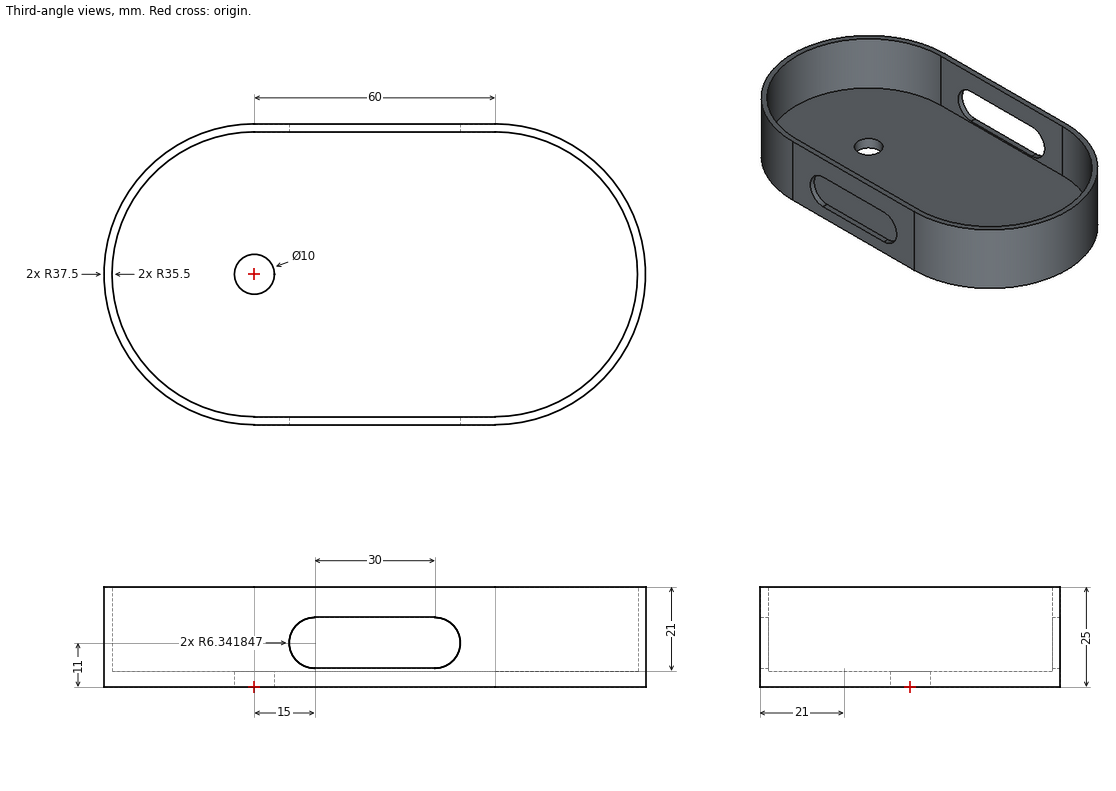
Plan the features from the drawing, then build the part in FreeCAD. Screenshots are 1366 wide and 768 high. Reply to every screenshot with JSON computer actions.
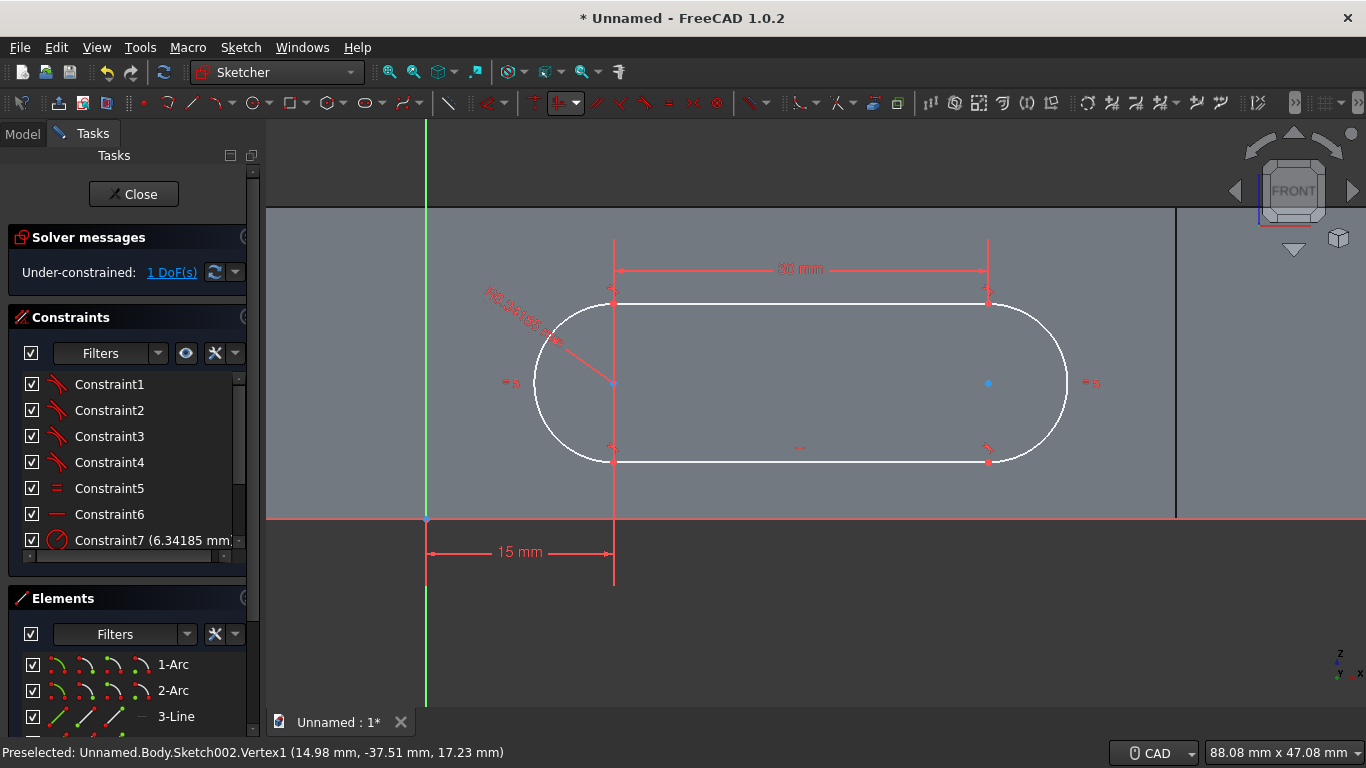
{"action": "left_click", "coordinate": [614, 383]}
{"action": "left_click", "coordinate": [392, 451]}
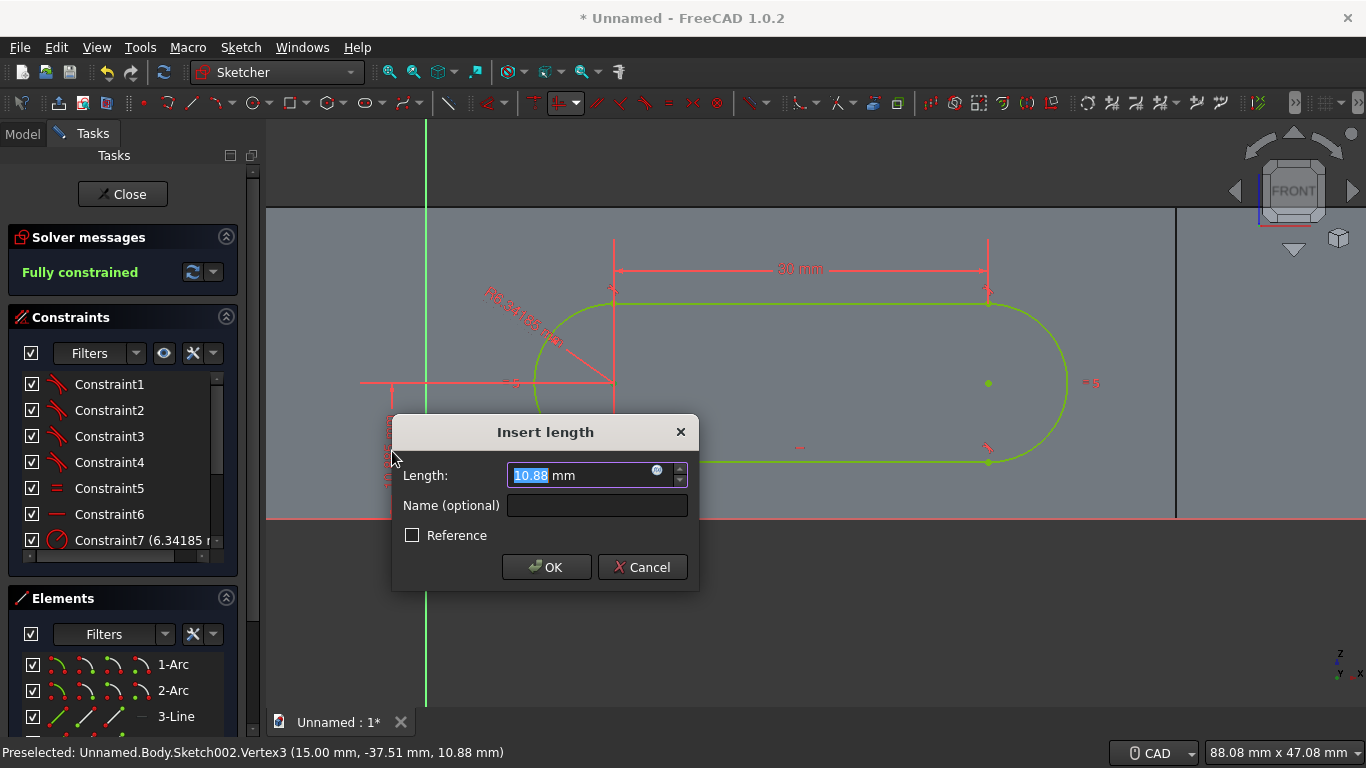
{"action": "type", "text": "11"}
{"action": "key", "text": "Return"}
{"action": "key", "text": "Escape"}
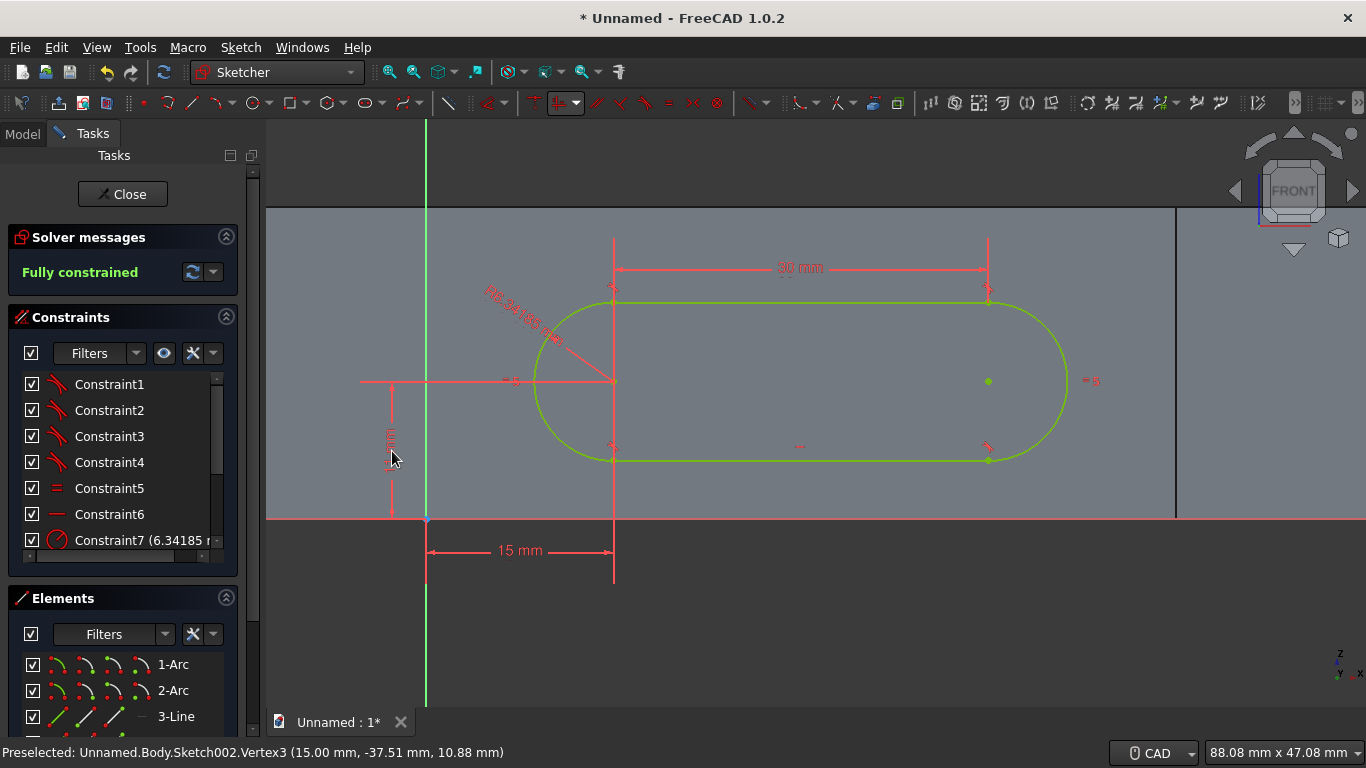
{"action": "left_click", "coordinate": [123, 194]}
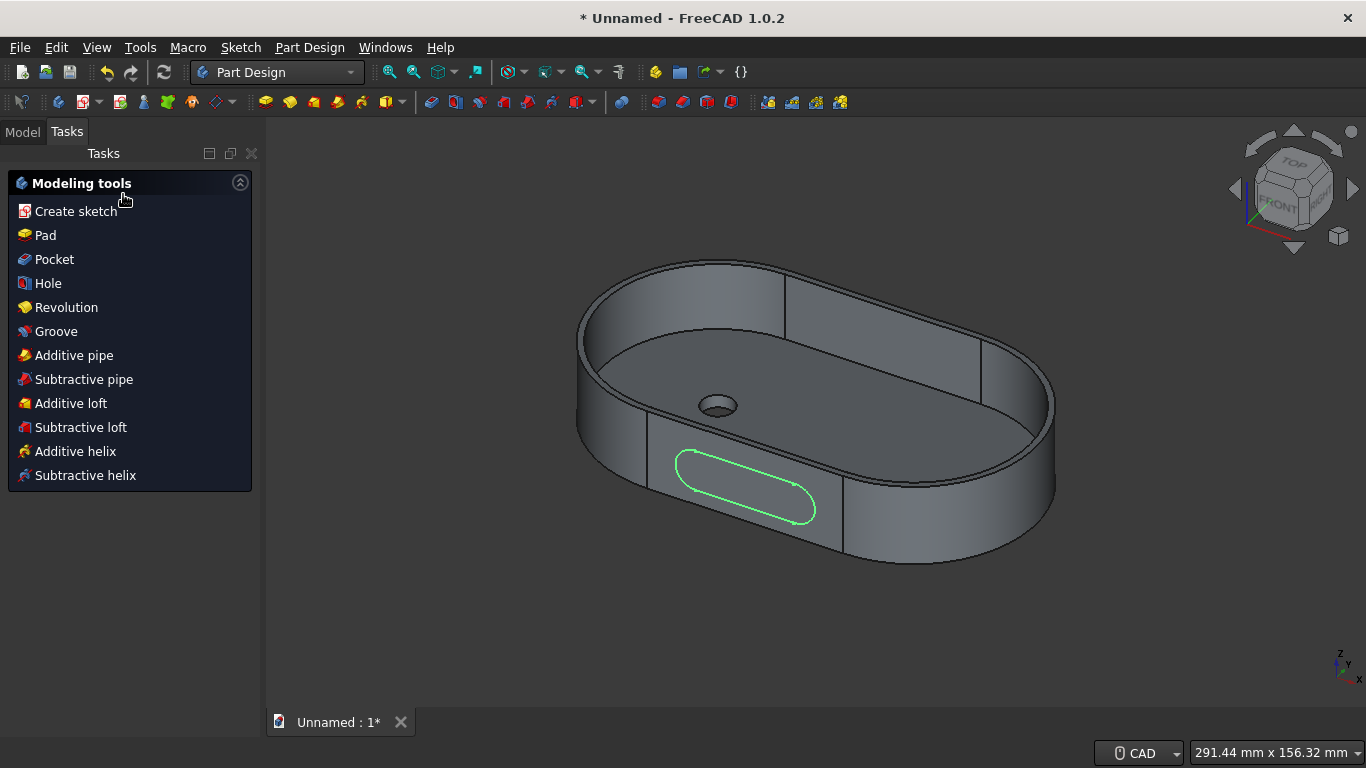
{"action": "left_click", "coordinate": [432, 102]}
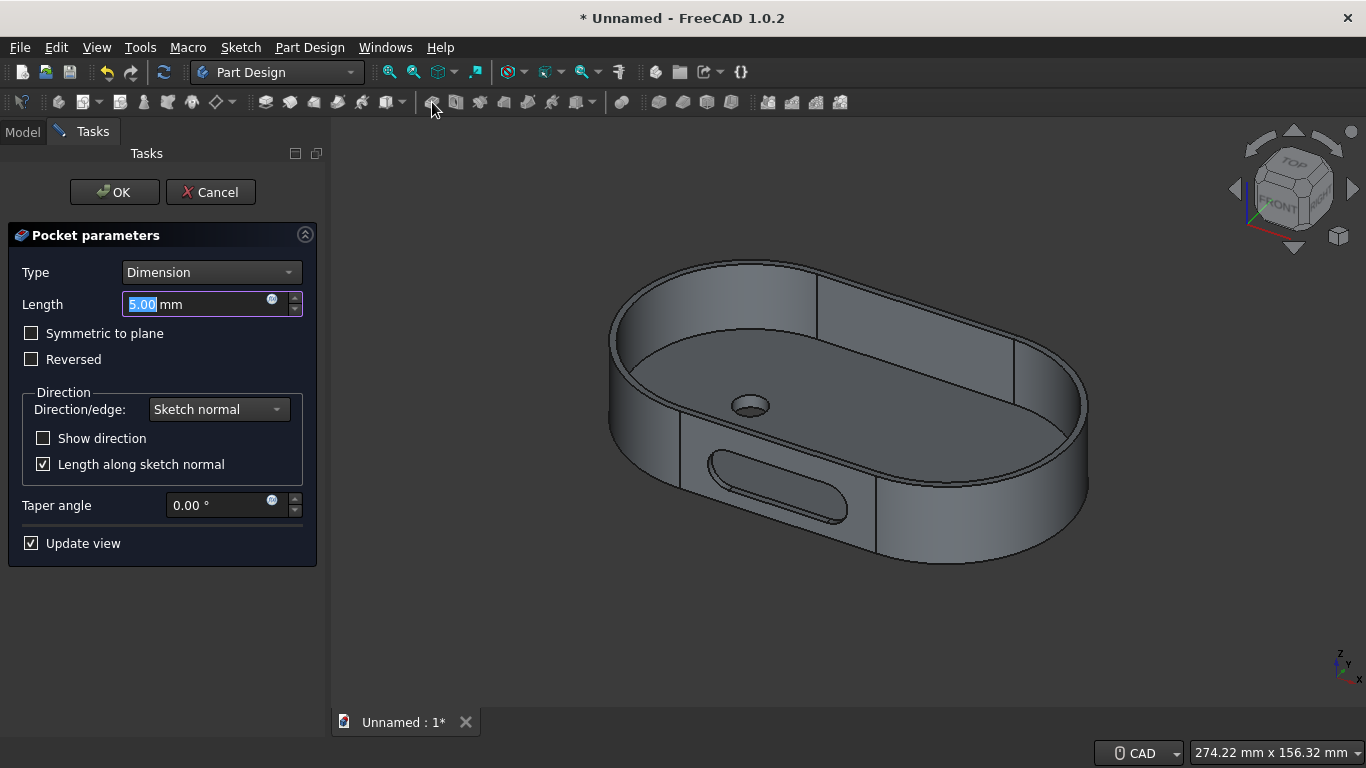
{"action": "type", "text": "21"}
{"action": "key", "text": "Tab"}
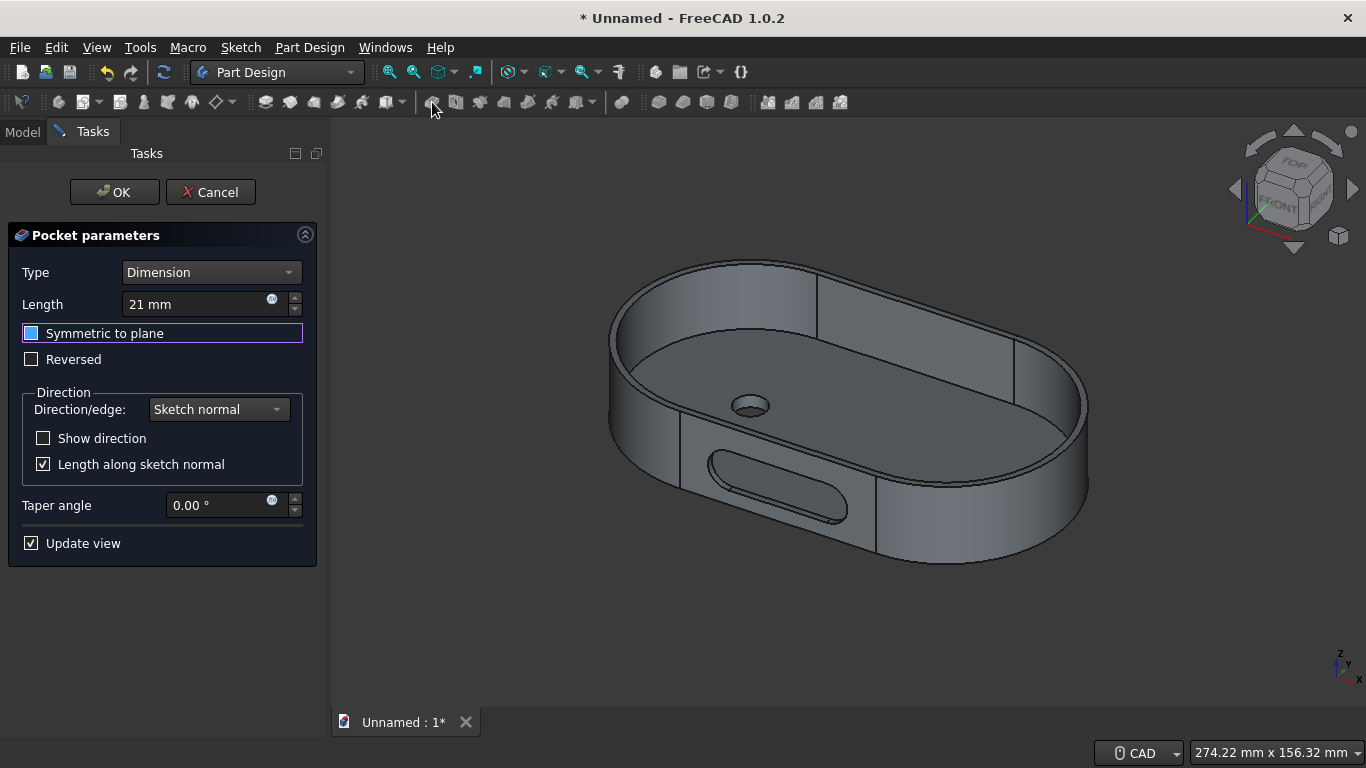
{"action": "left_click", "coordinate": [115, 192]}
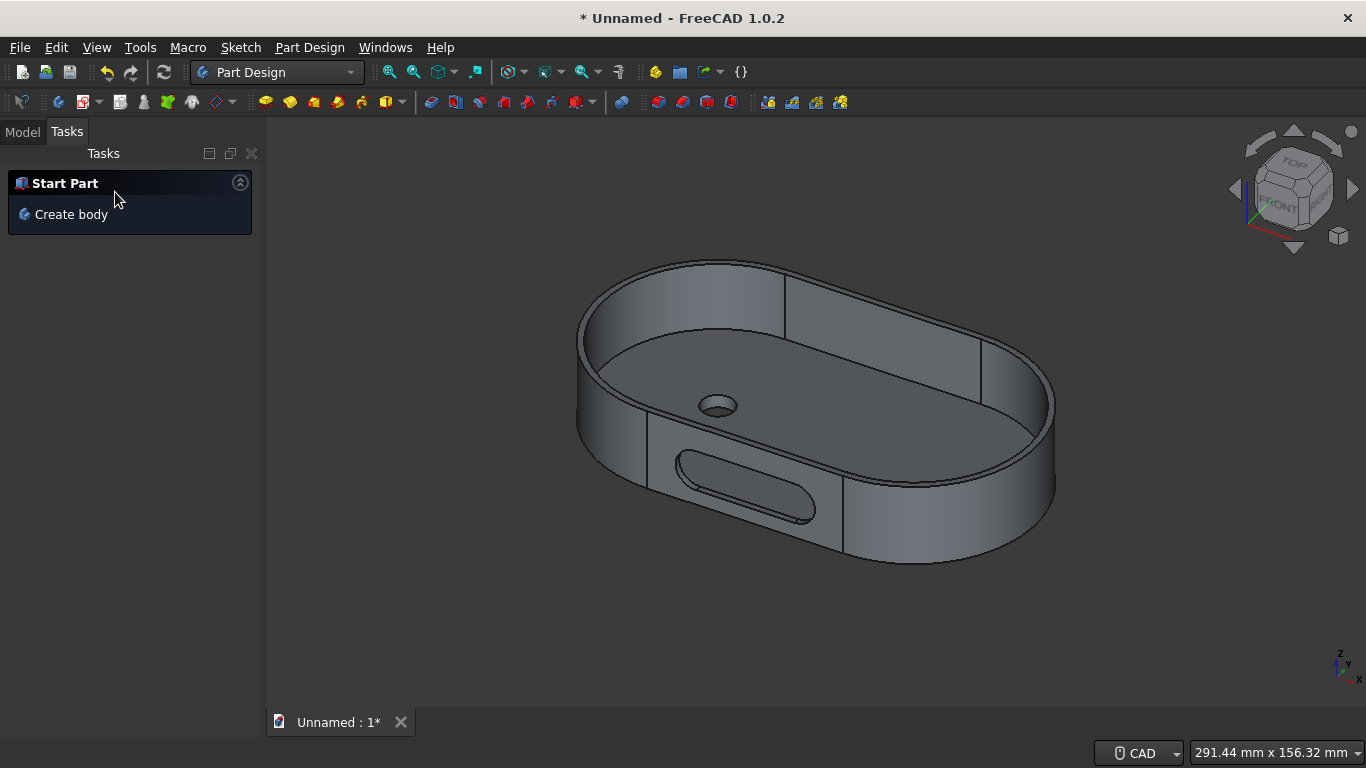
{"action": "left_click", "coordinate": [23, 131]}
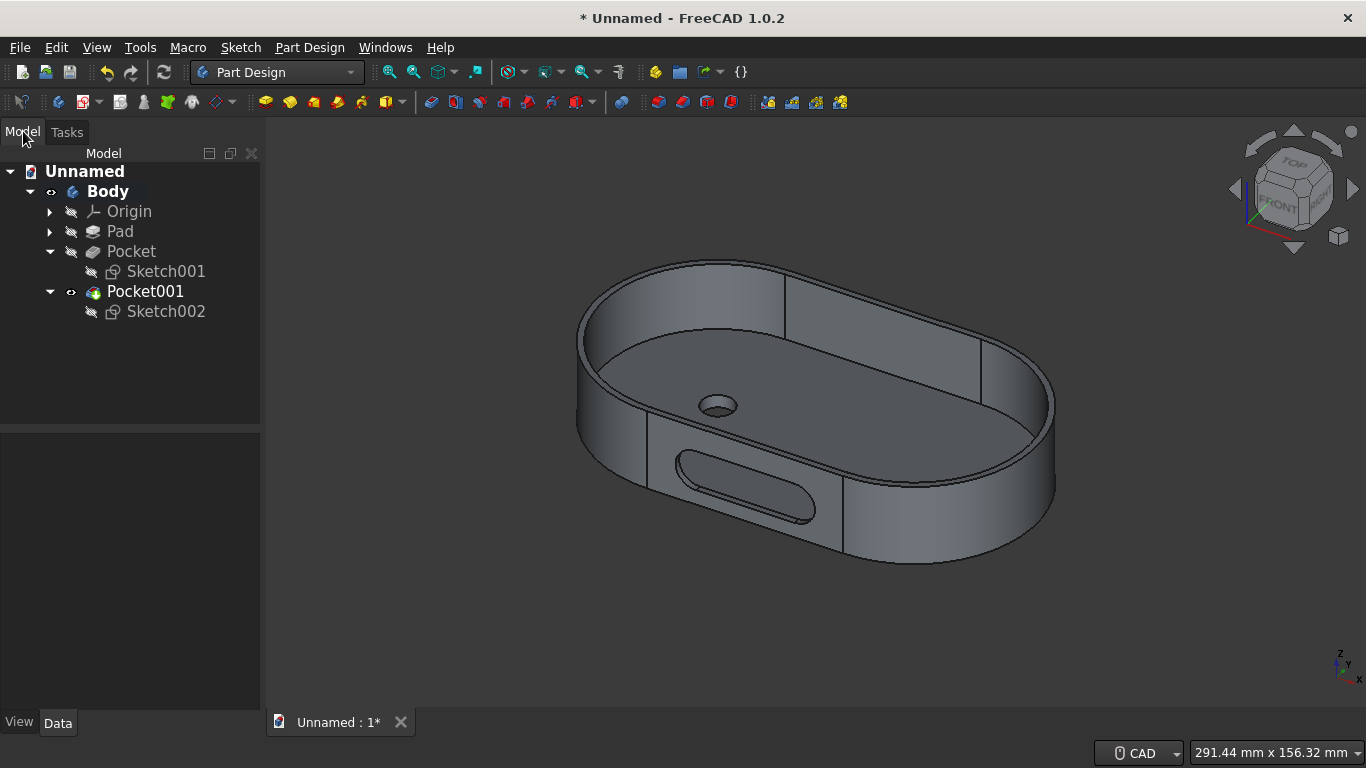
{"action": "left_click", "coordinate": [116, 292]}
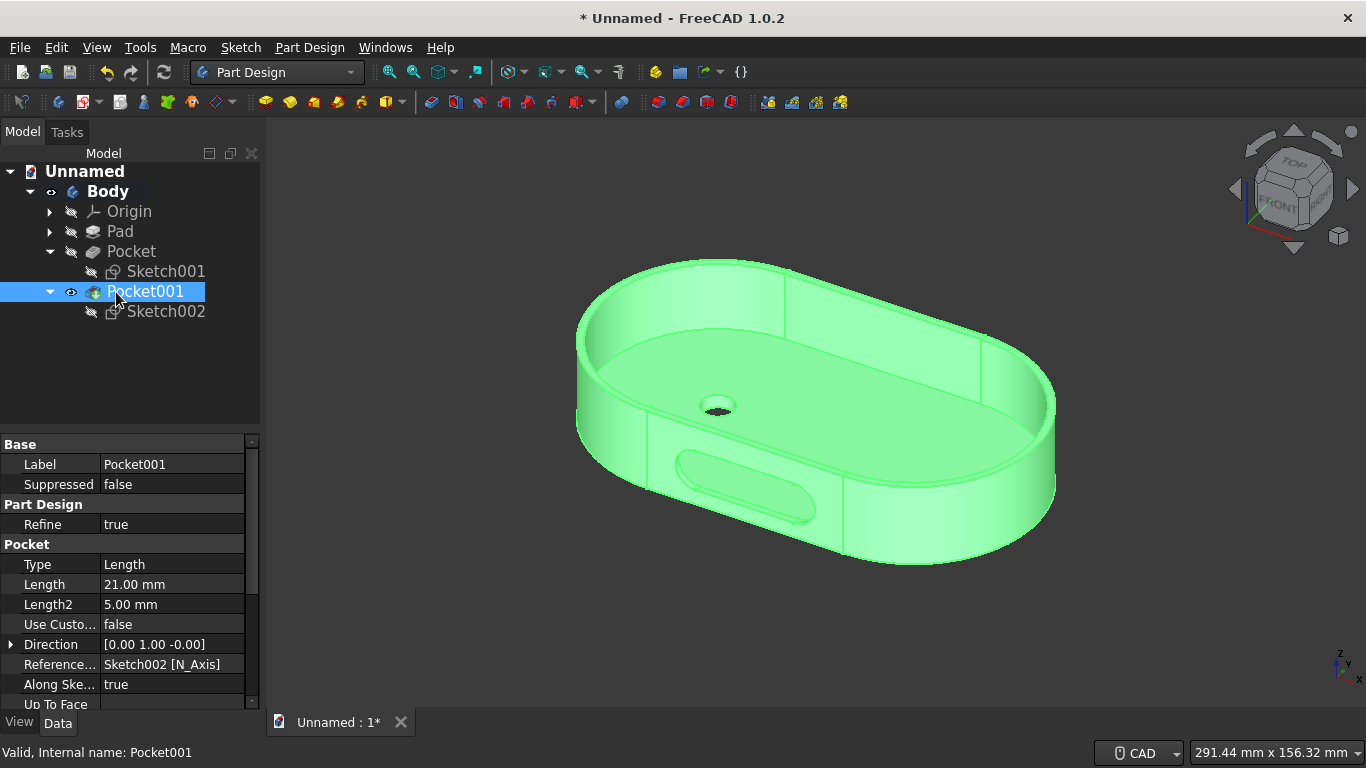
{"action": "left_click", "coordinate": [768, 102]}